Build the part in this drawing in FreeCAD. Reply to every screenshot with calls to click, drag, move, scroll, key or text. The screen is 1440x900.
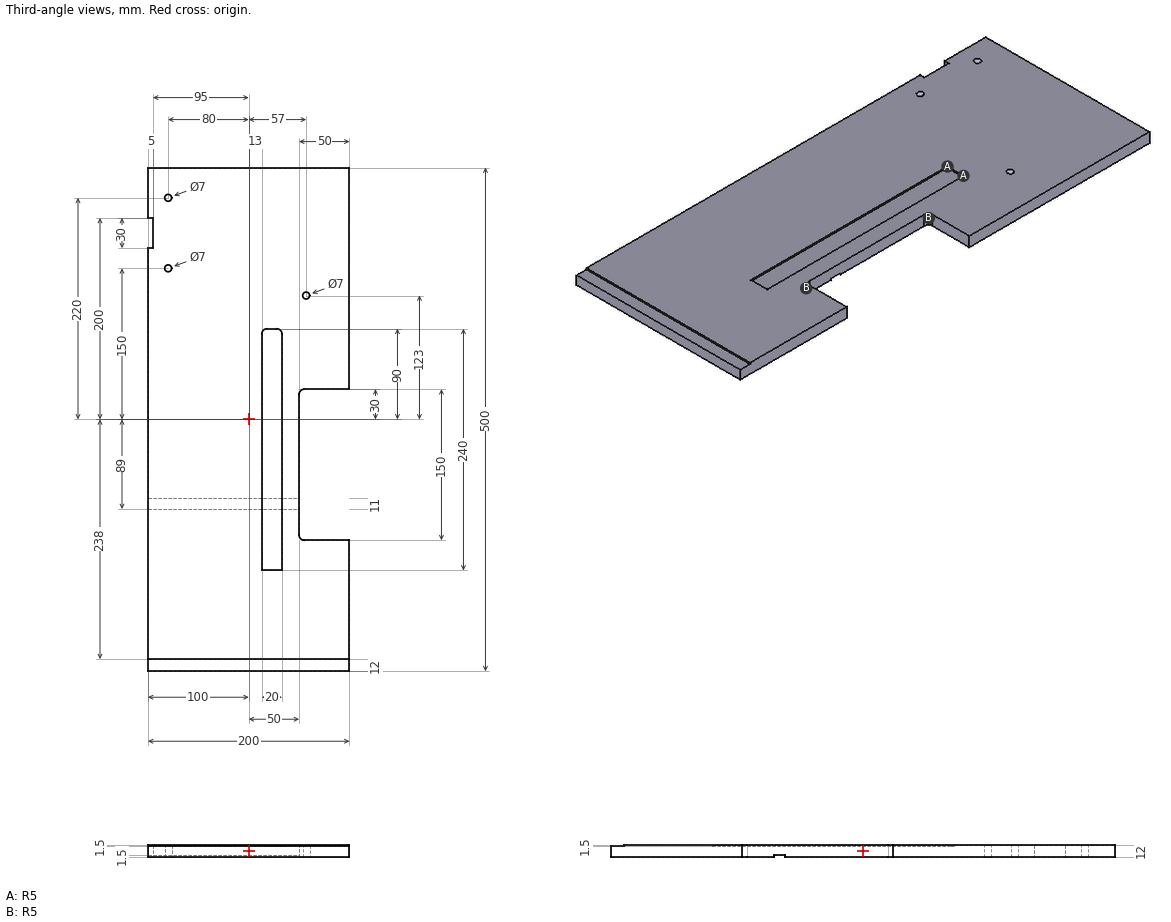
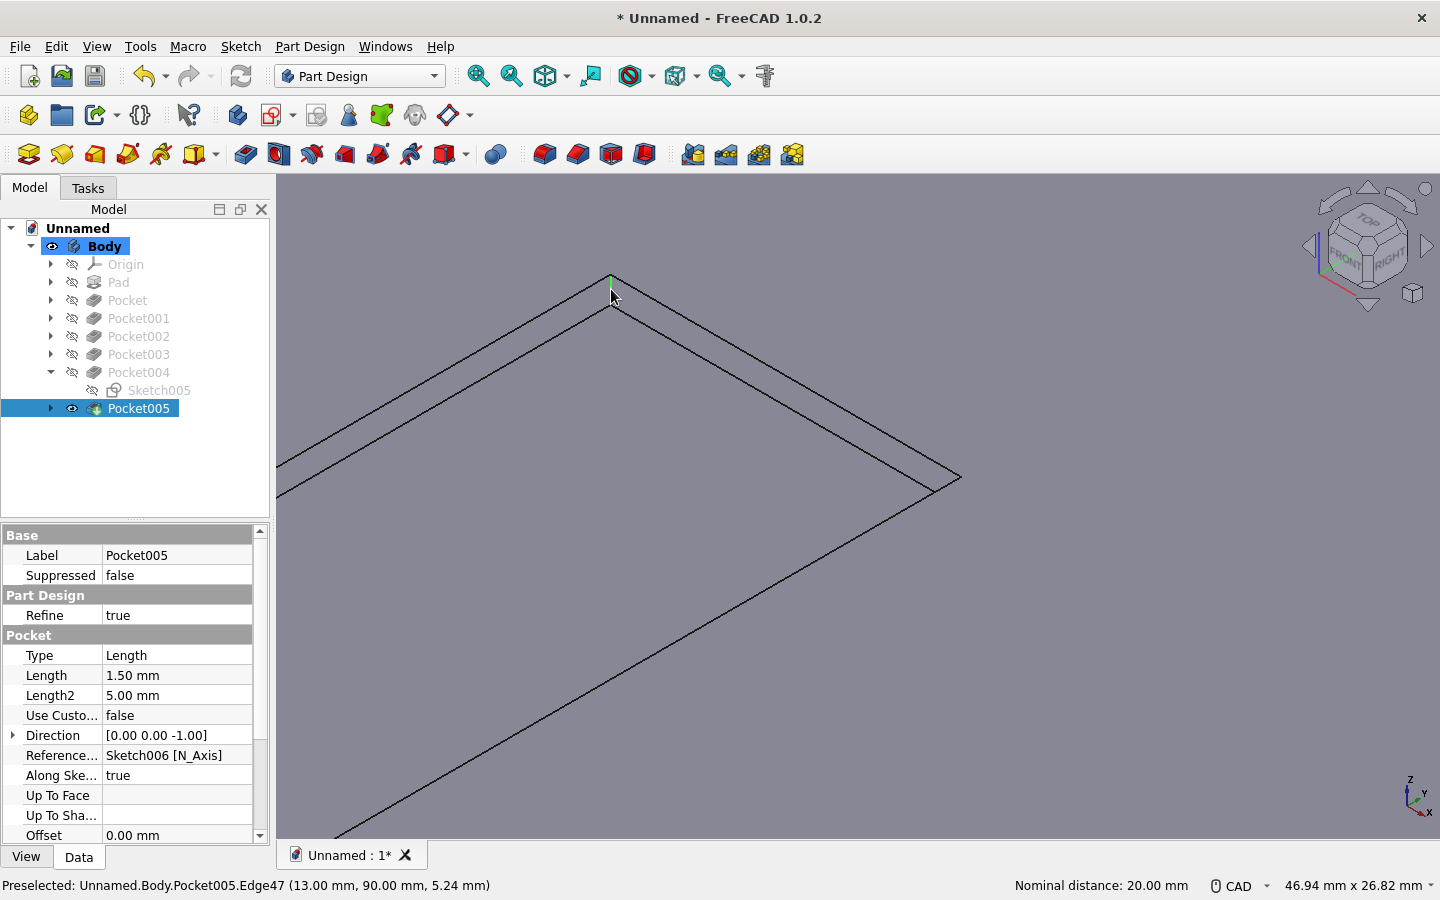
click(545, 154)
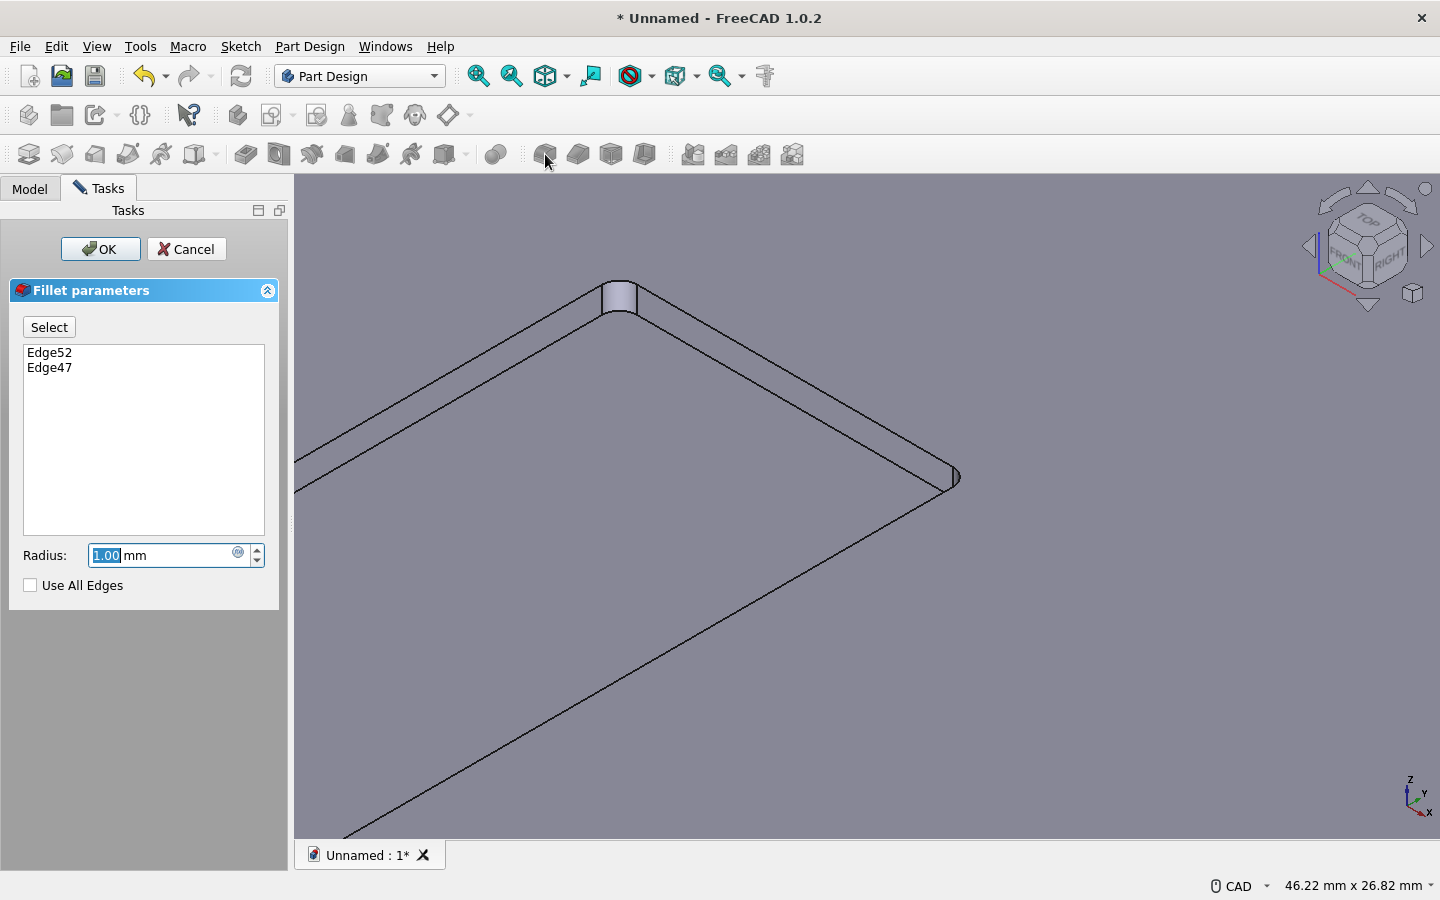
text(5)
key(Tab)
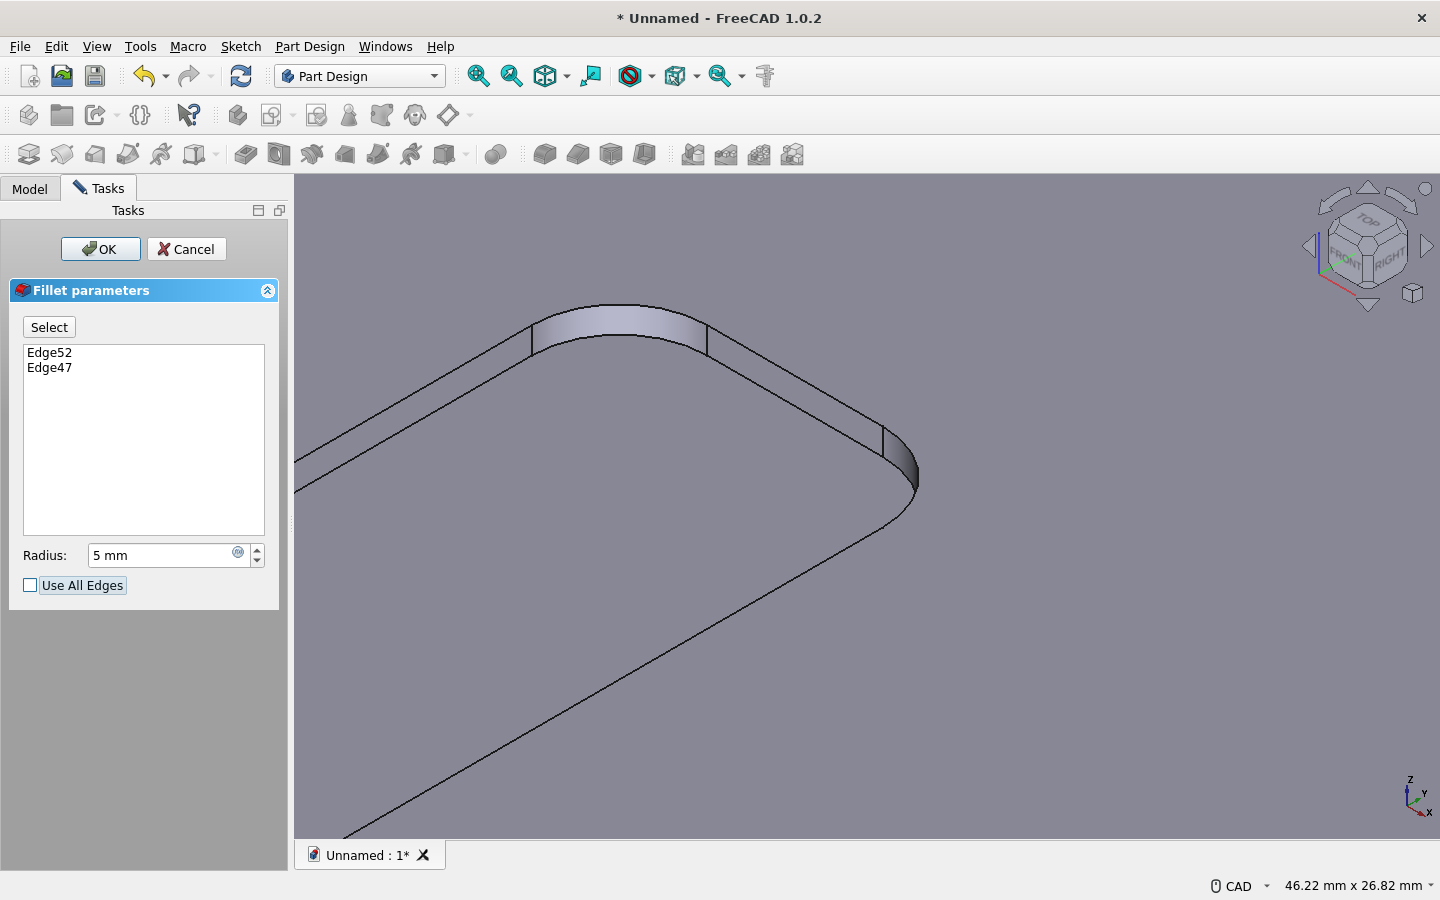
click(101, 249)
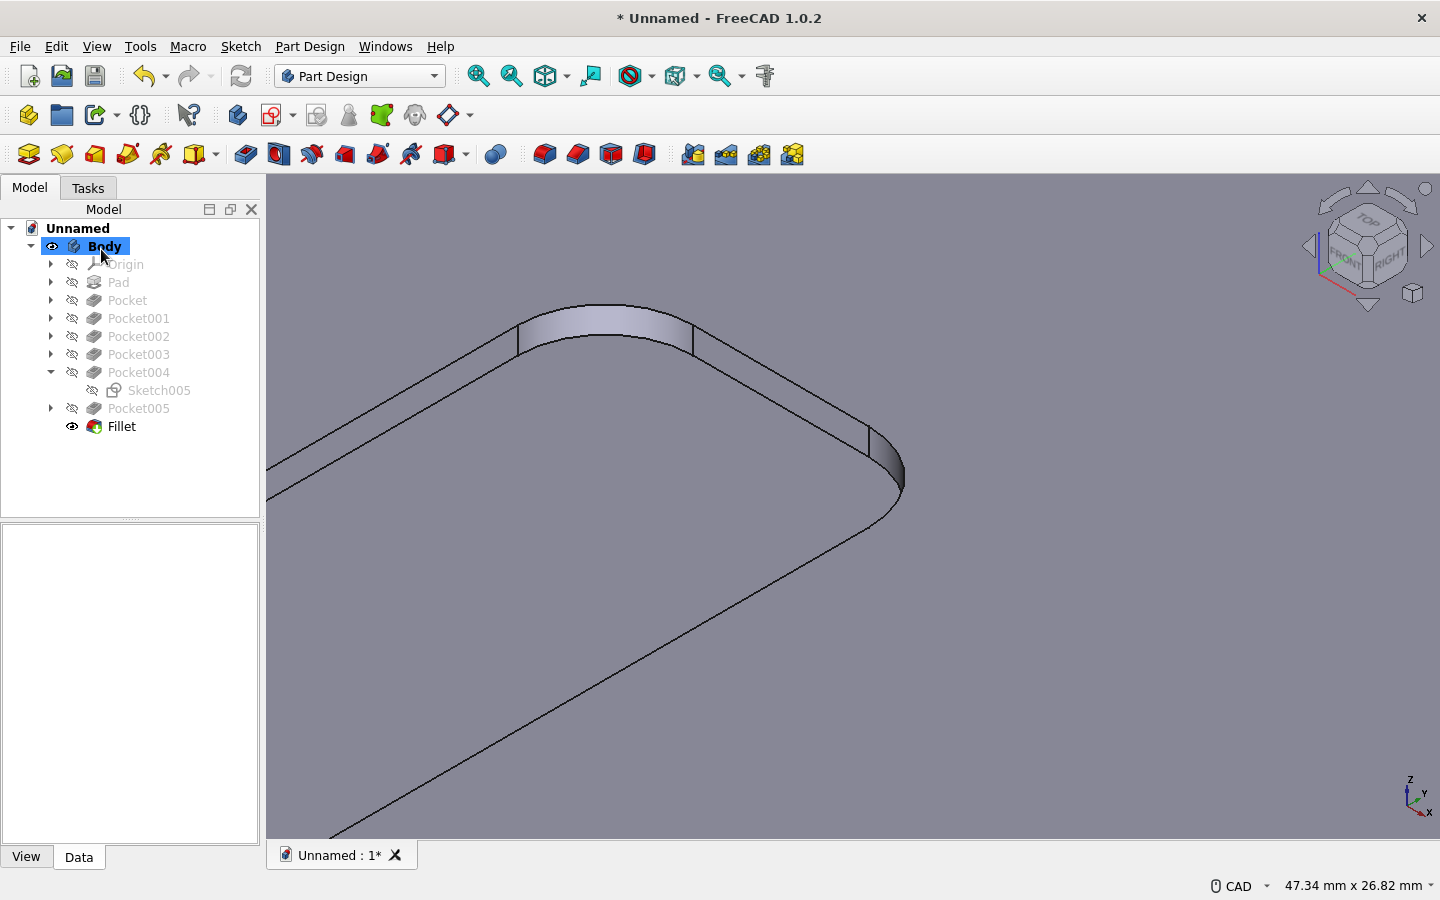
click(479, 76)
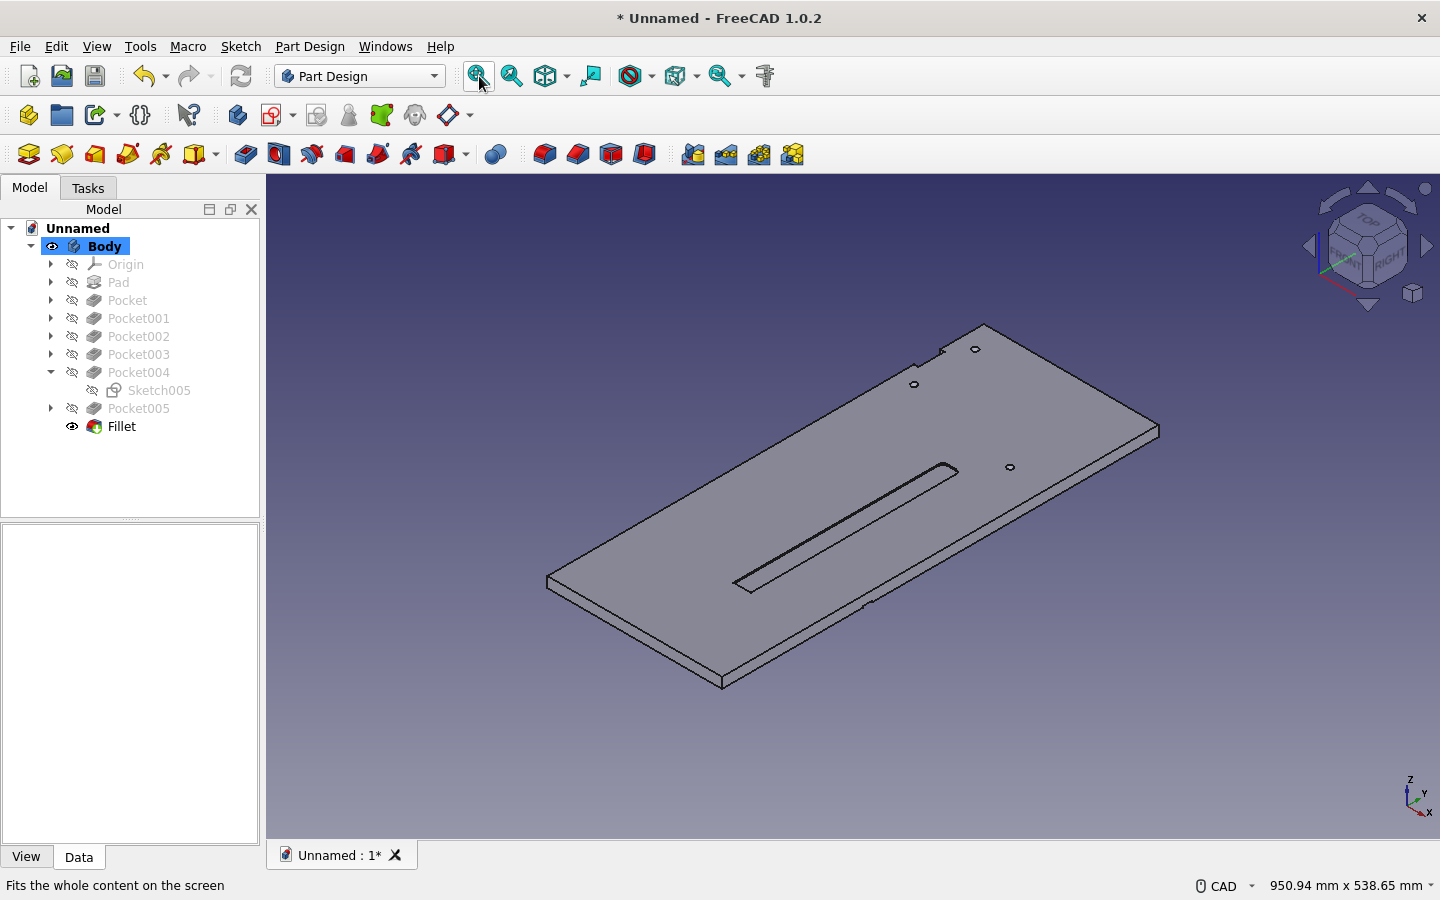
key(5)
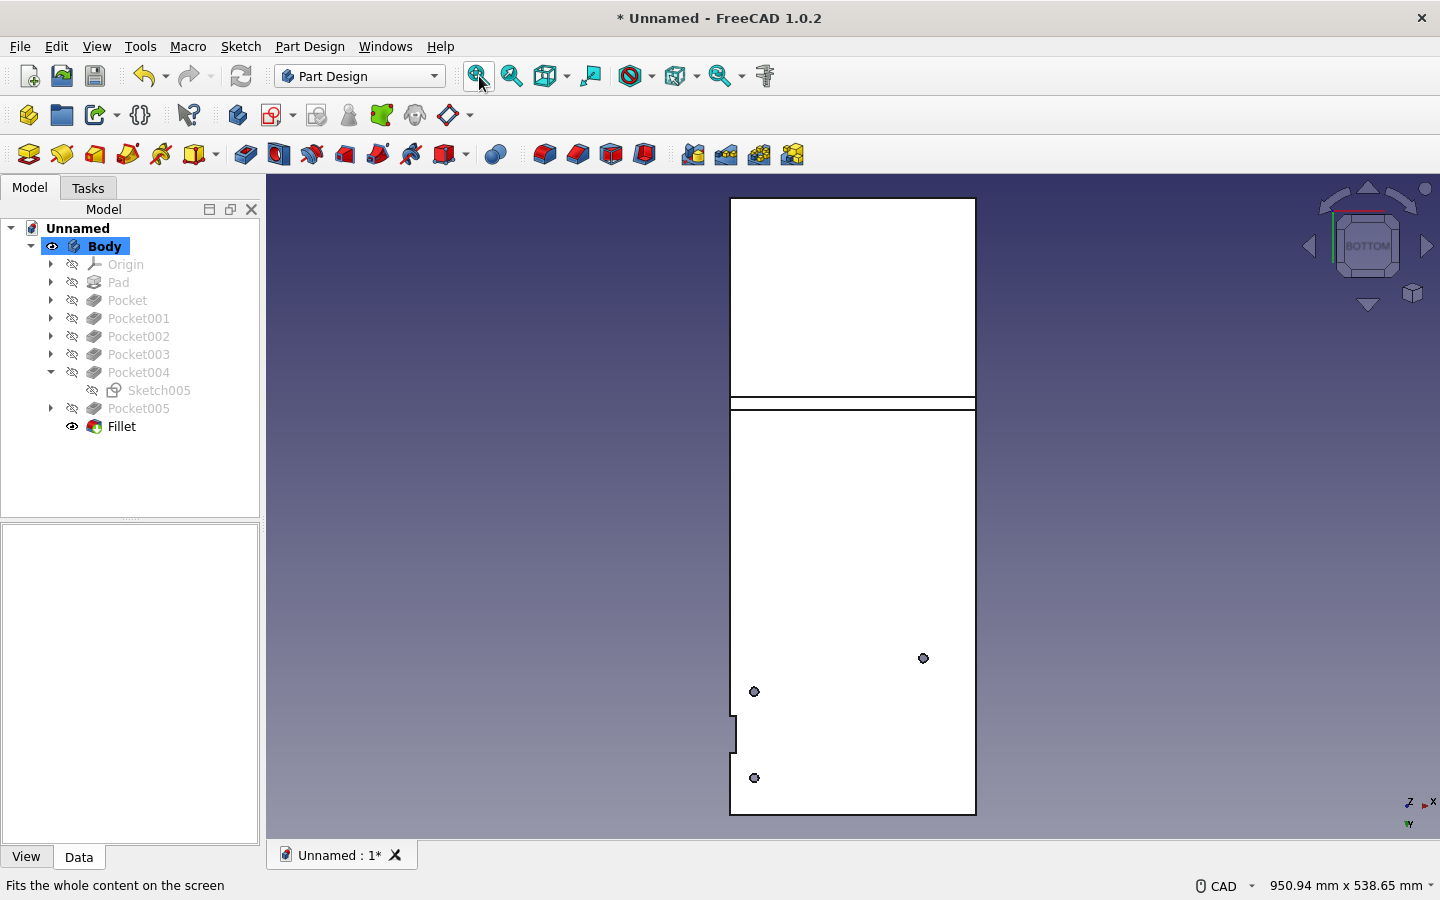
click(853, 554)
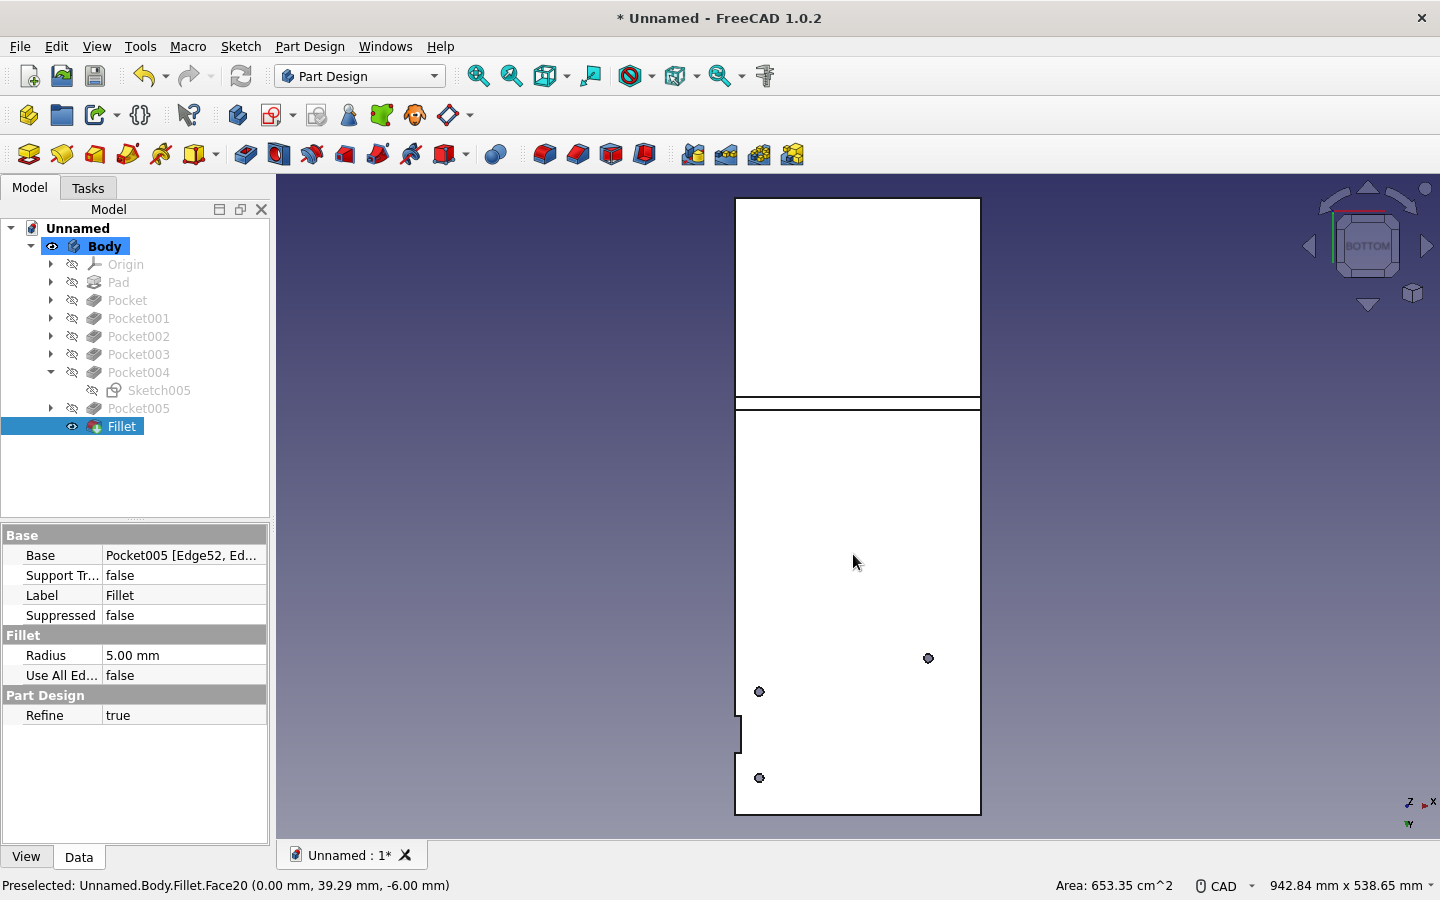
click(270, 116)